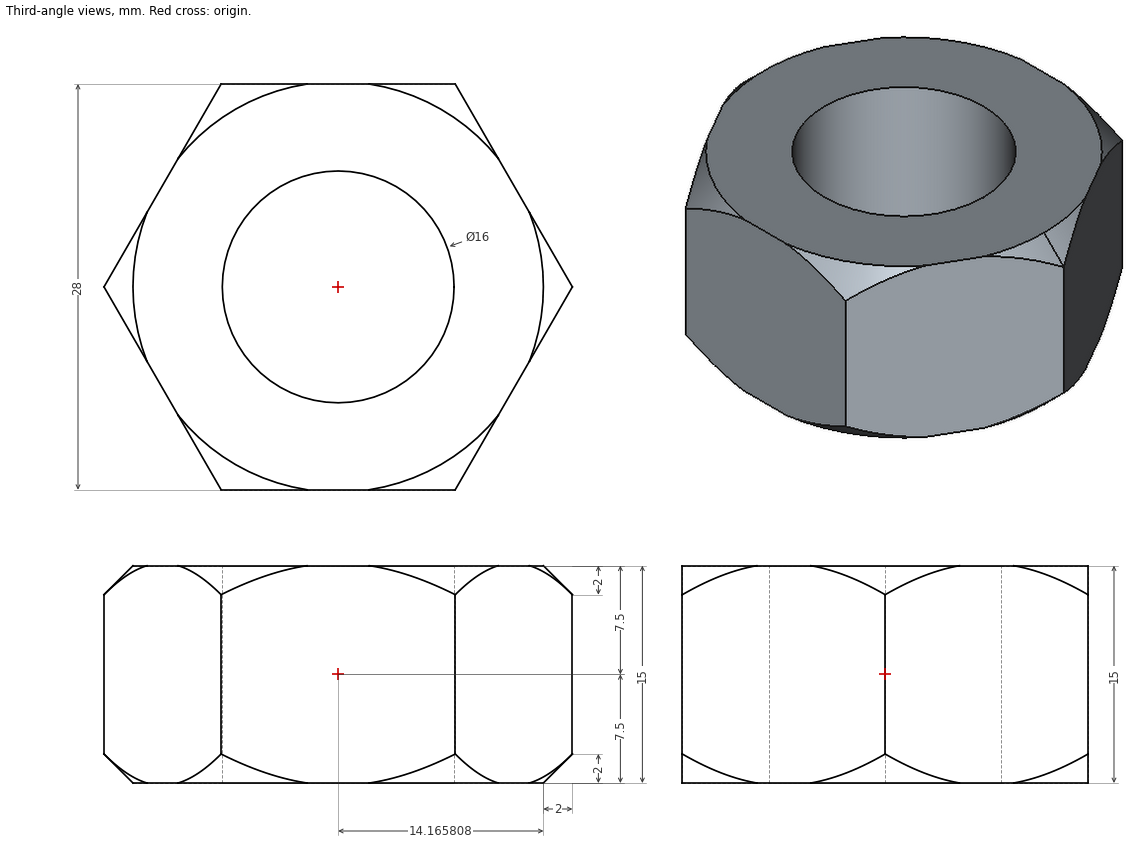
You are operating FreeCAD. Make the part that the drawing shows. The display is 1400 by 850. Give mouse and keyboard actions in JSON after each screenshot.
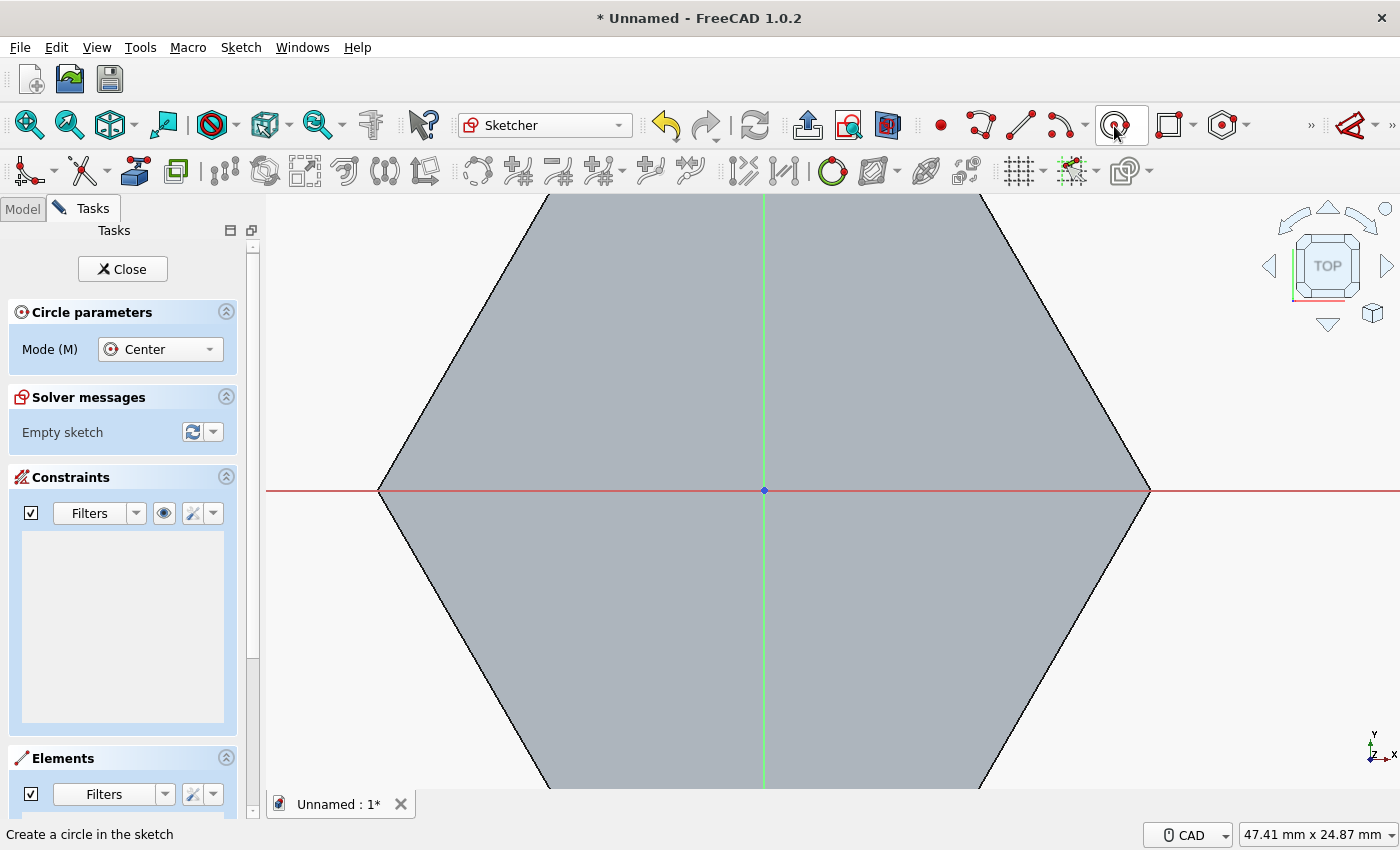
{"action": "left_click", "coordinate": [764, 491]}
{"action": "mouse_move", "coordinate": [900, 355]}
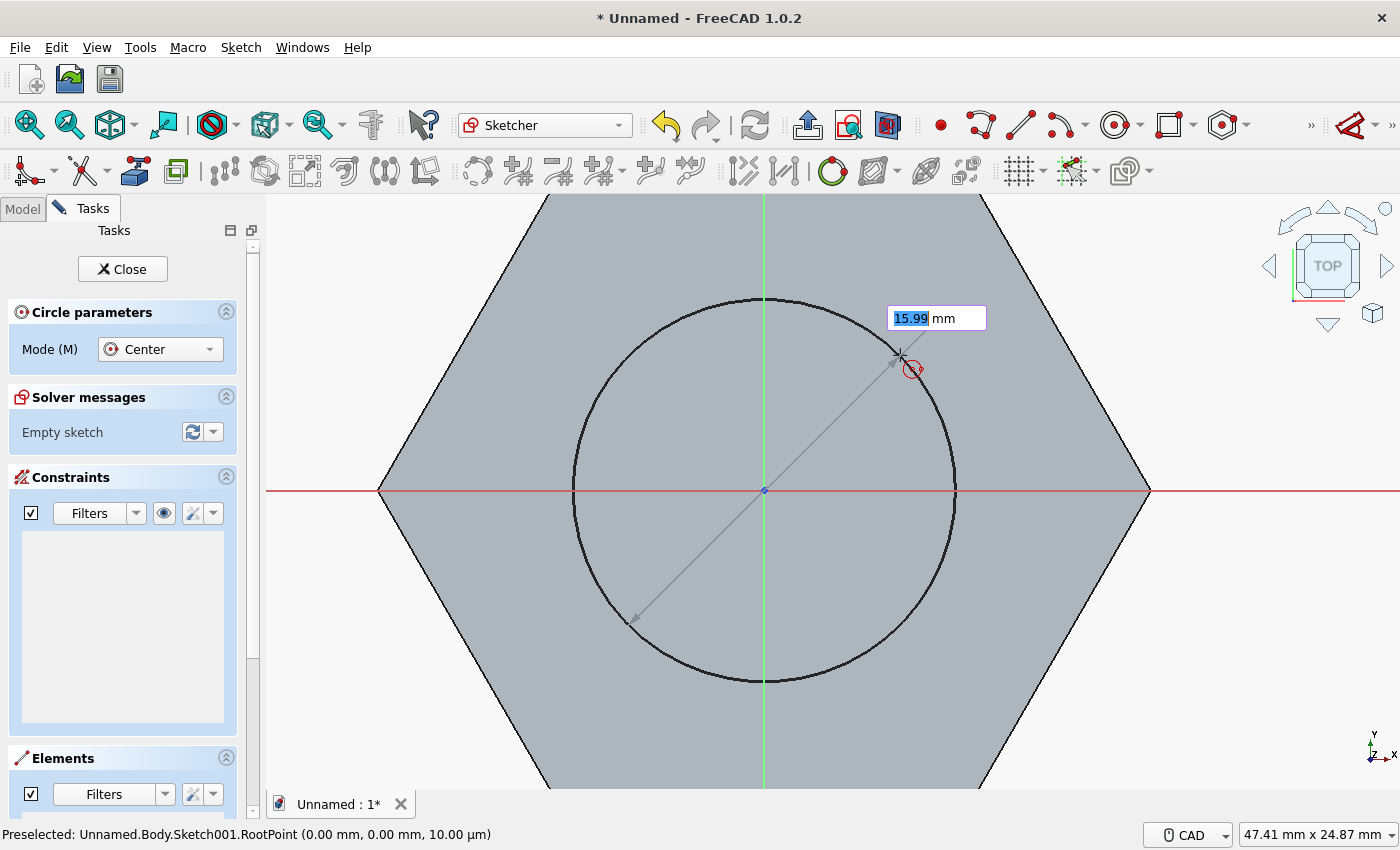
{"action": "type", "text": "16"}
{"action": "key", "text": "Return"}
{"action": "key", "text": "Escape"}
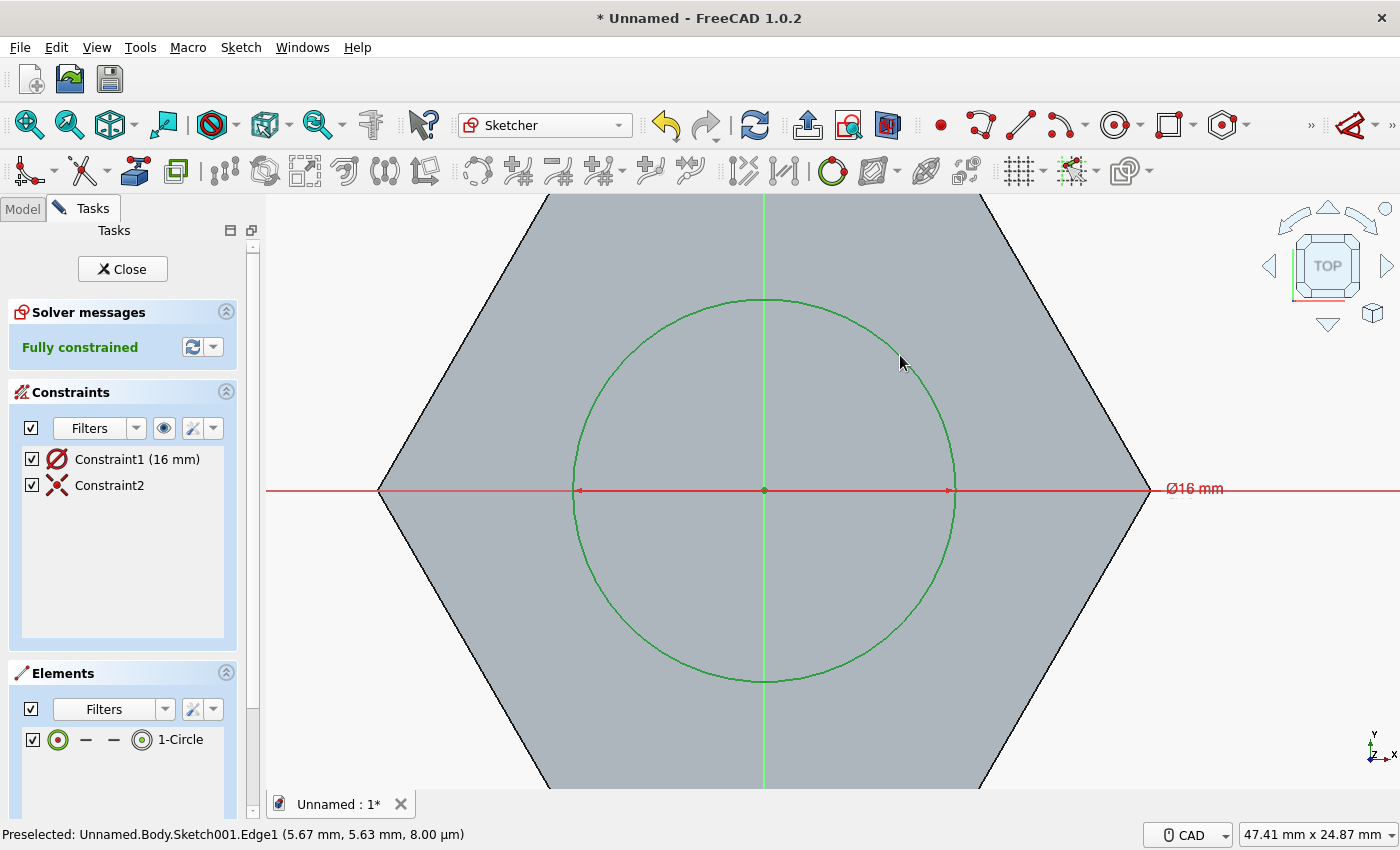
{"action": "left_click", "coordinate": [123, 269]}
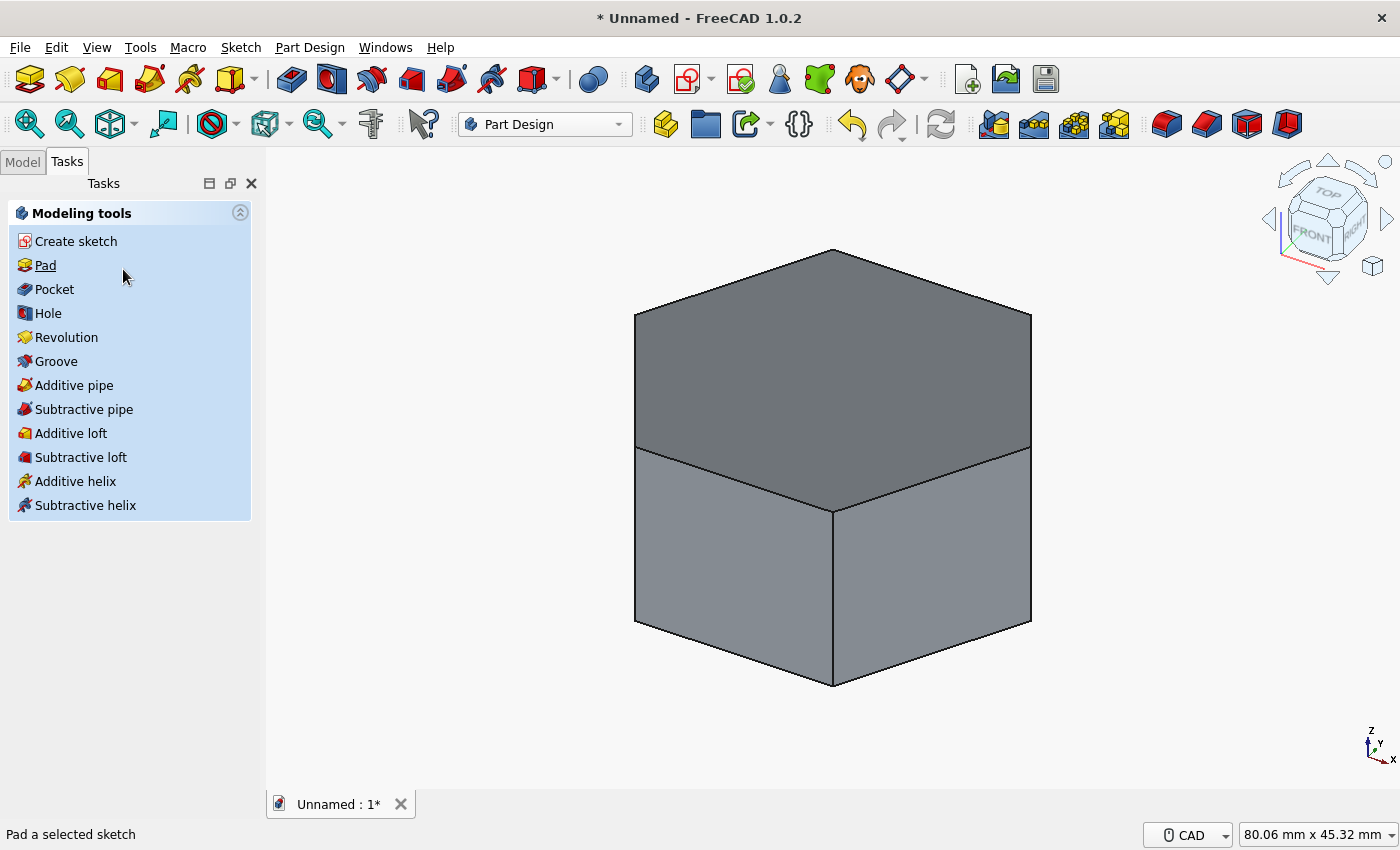
{"action": "left_click", "coordinate": [292, 80]}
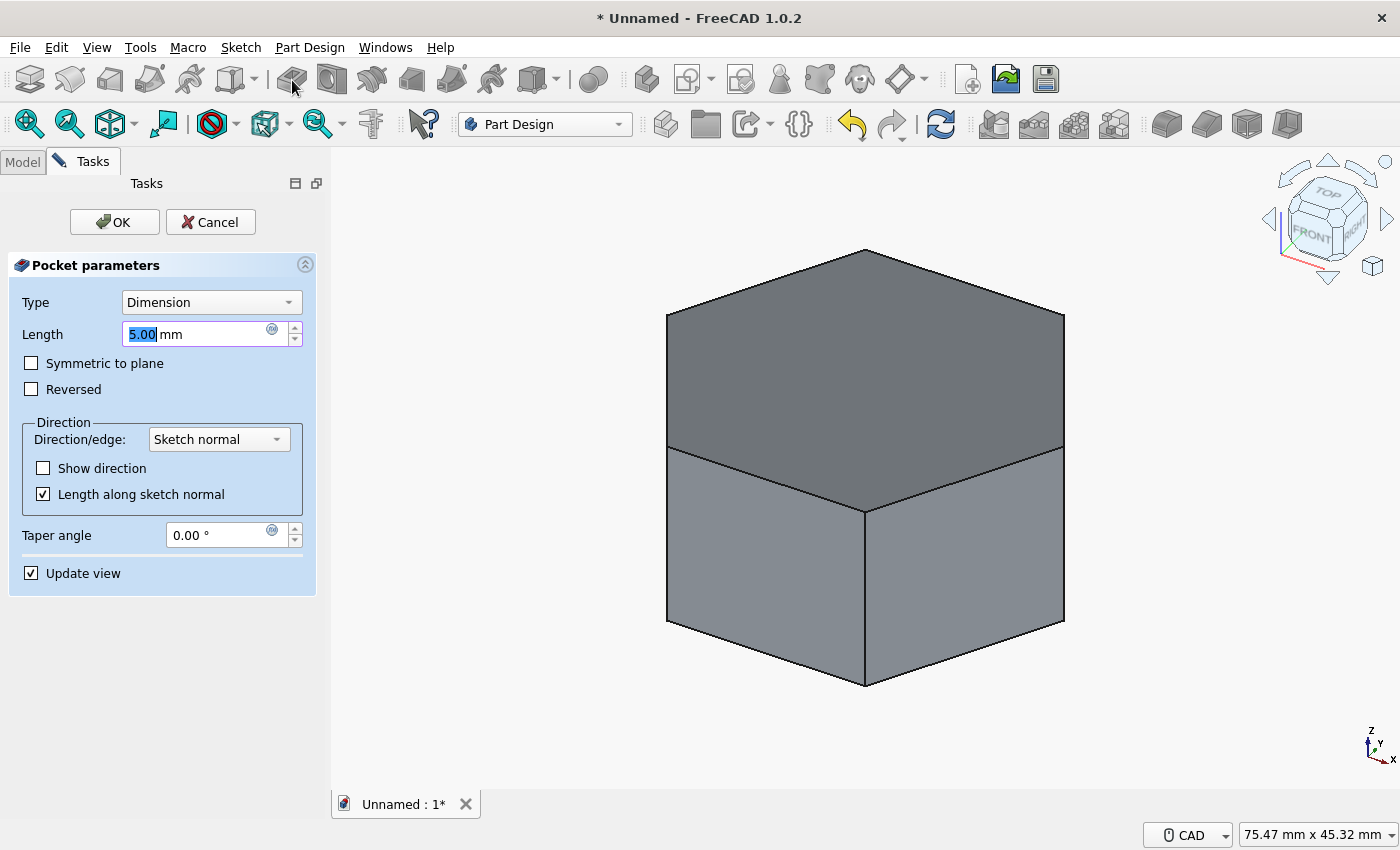
{"action": "type", "text": "15"}
{"action": "key", "text": "Tab"}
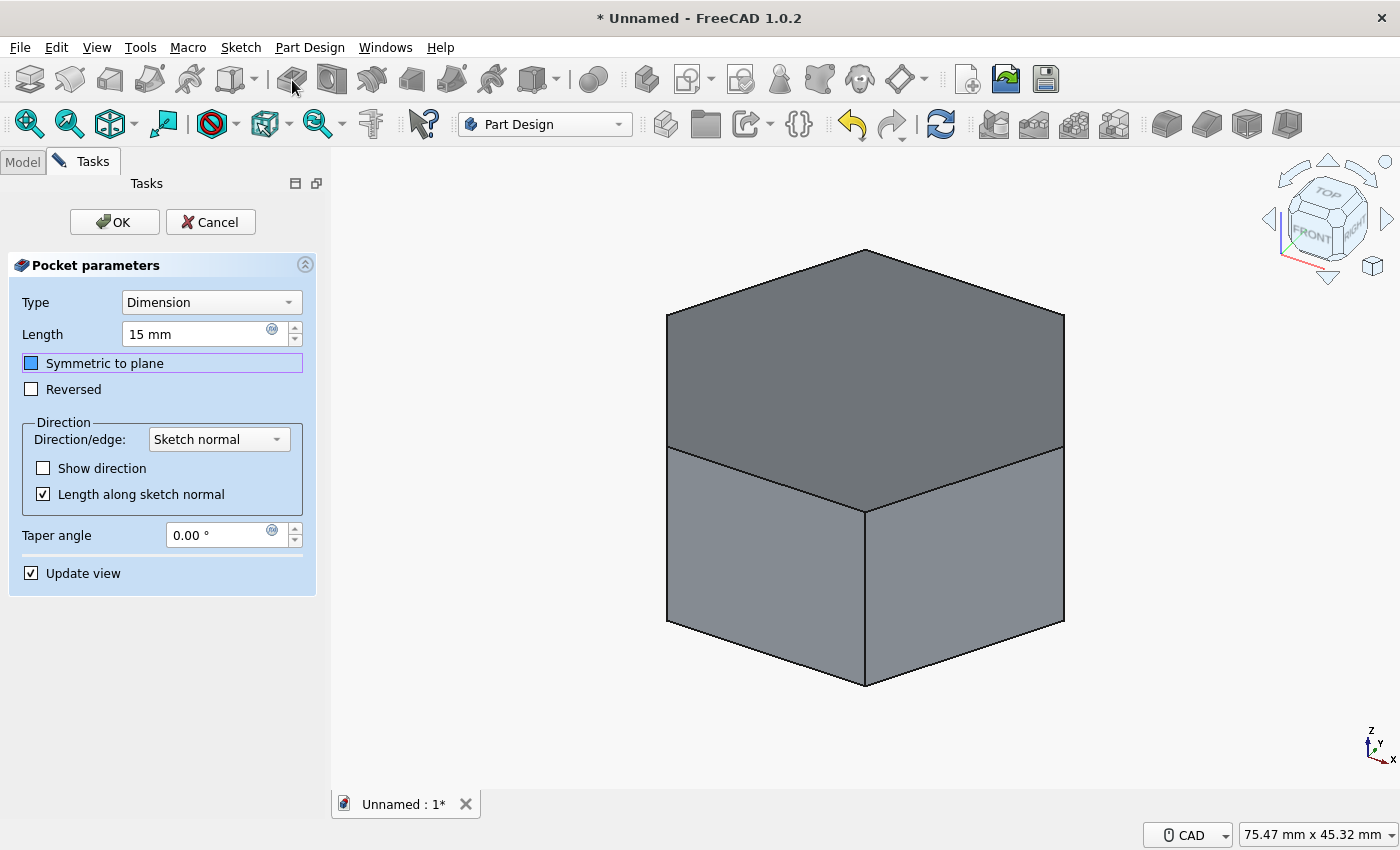
{"action": "left_click", "coordinate": [30, 363]}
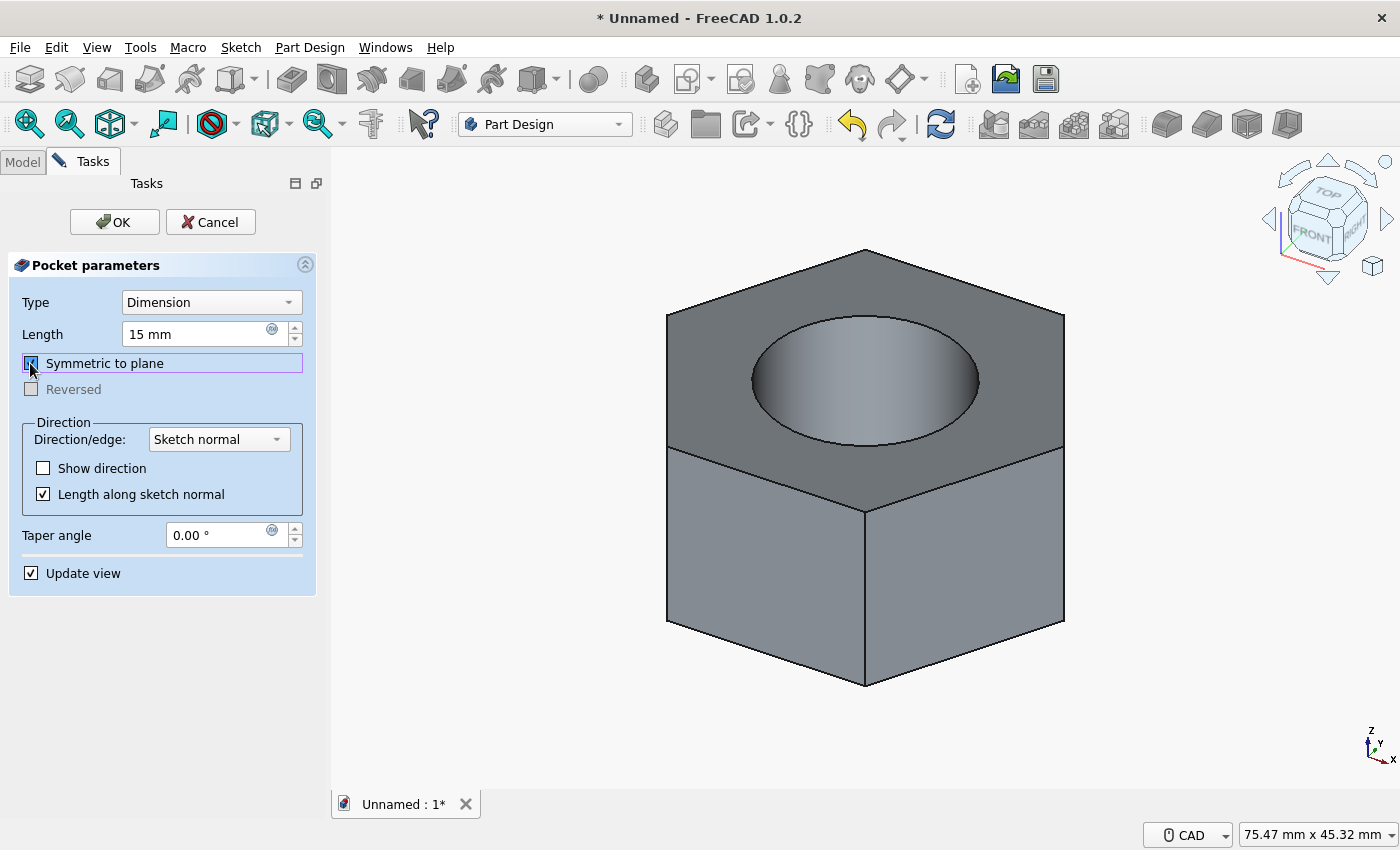
{"action": "left_click", "coordinate": [115, 222]}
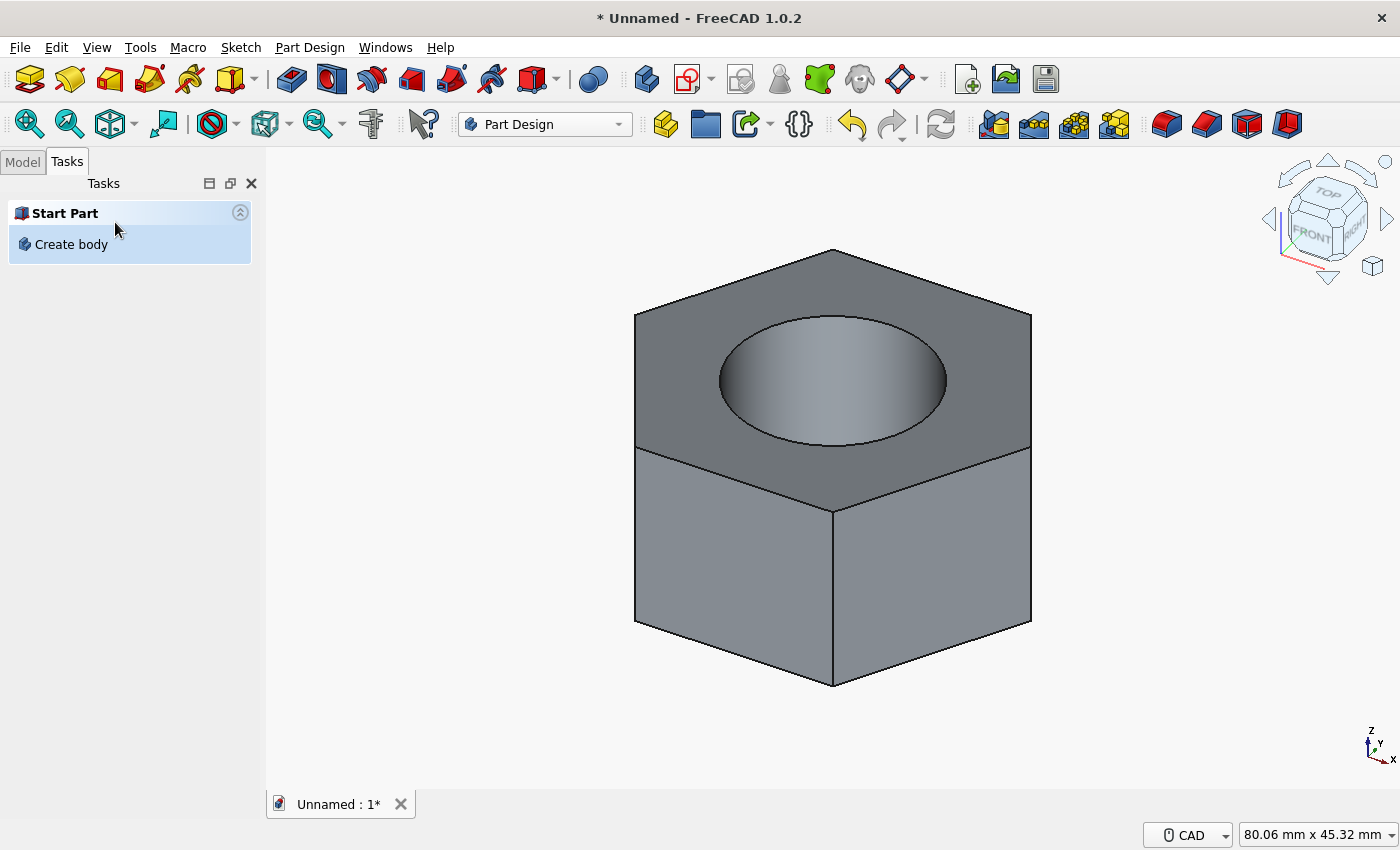
{"action": "left_click", "coordinate": [688, 80]}